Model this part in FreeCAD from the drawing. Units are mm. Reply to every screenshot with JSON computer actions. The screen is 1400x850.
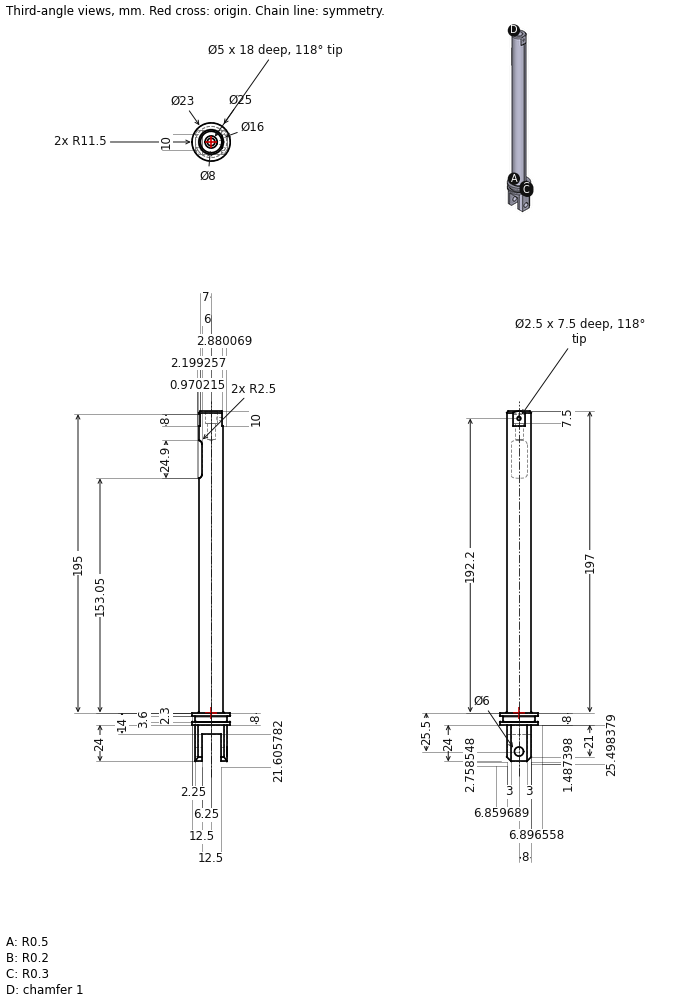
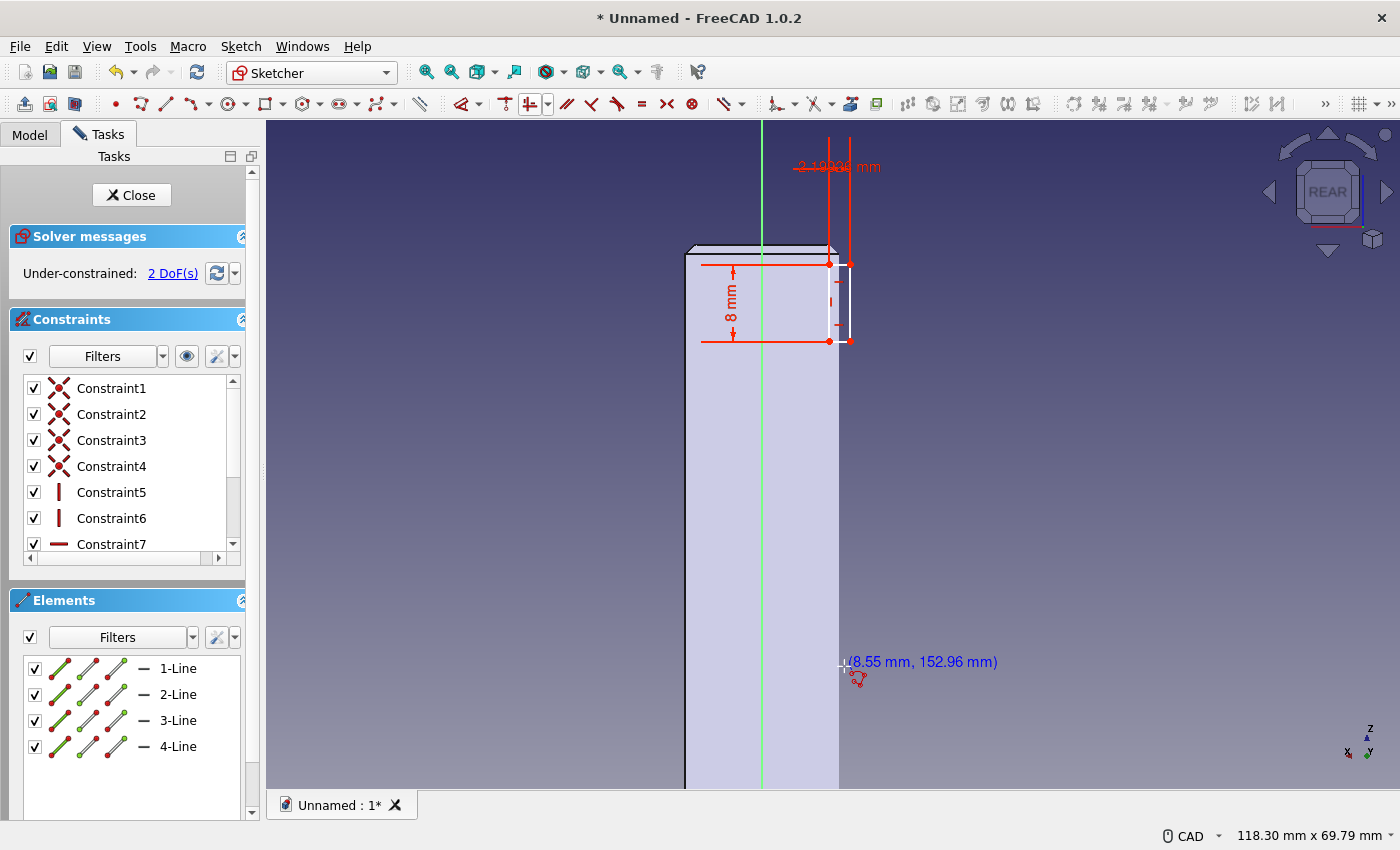
{"action": "scroll", "coordinate": [853, 666], "scroll_direction": "up", "scroll_amount": 3}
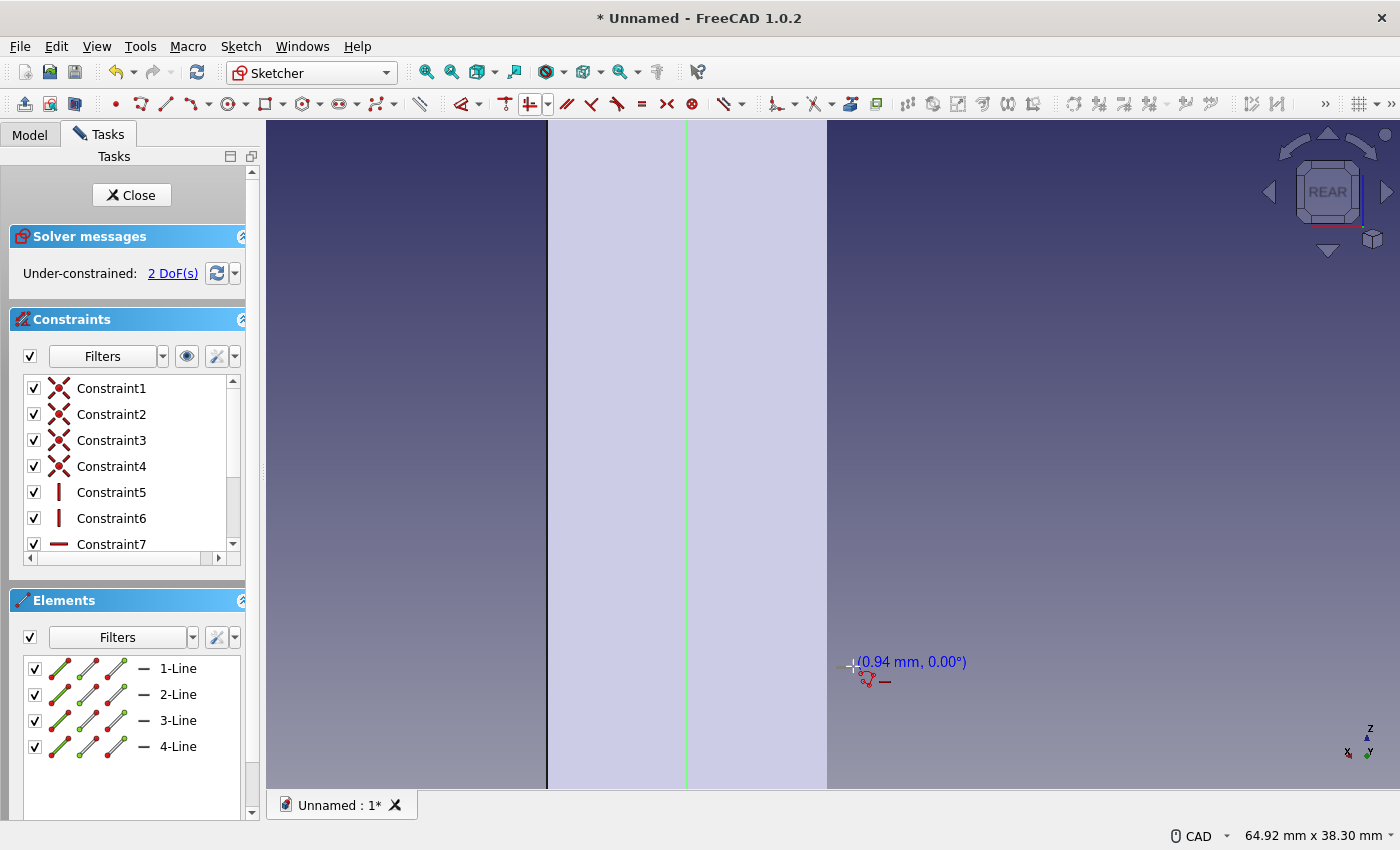
{"action": "left_click", "coordinate": [852, 665]}
{"action": "left_click", "coordinate": [852, 231]}
{"action": "left_click", "coordinate": [835, 231]}
{"action": "right_click", "coordinate": [835, 231]}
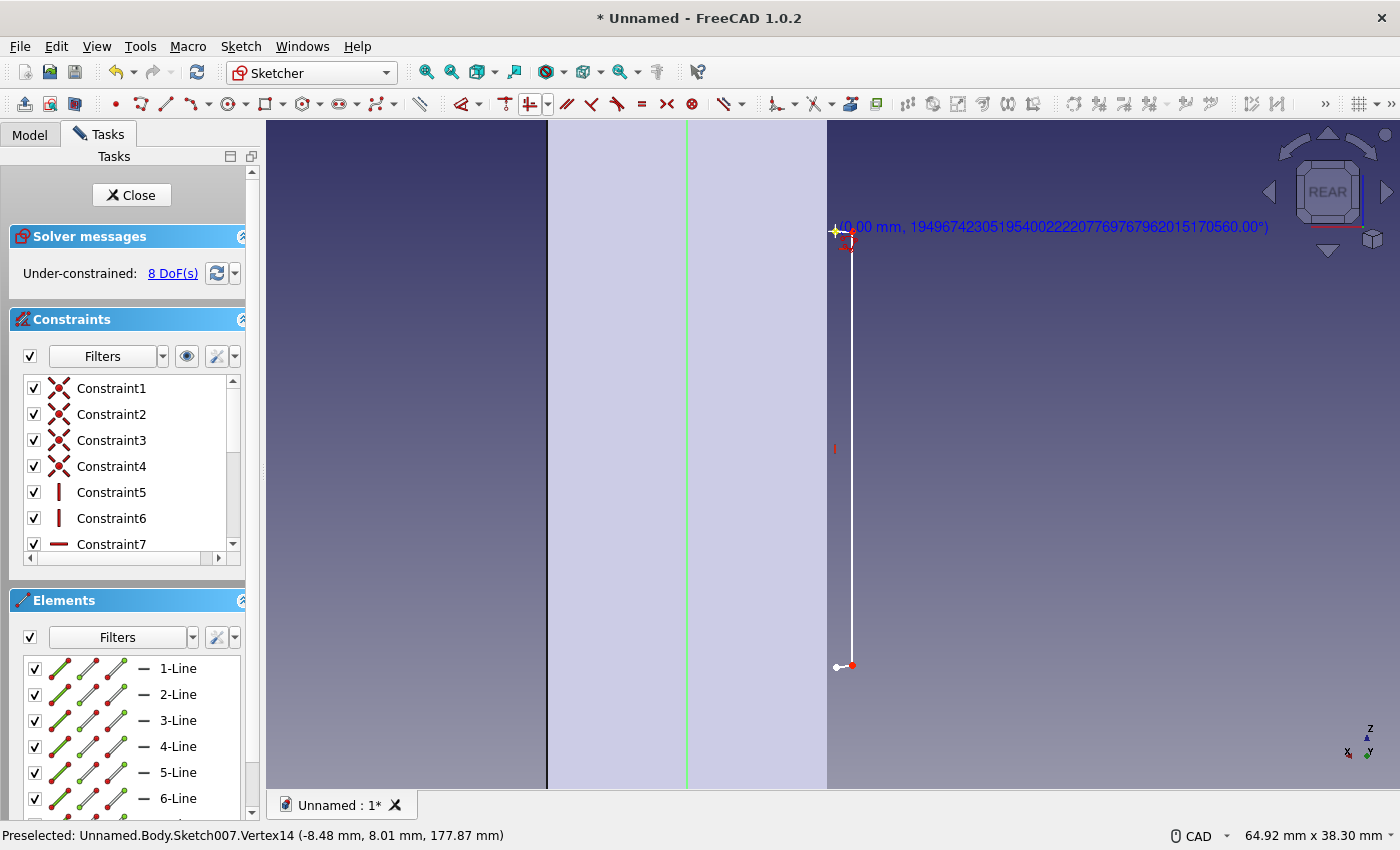
{"action": "left_click", "coordinate": [166, 104]}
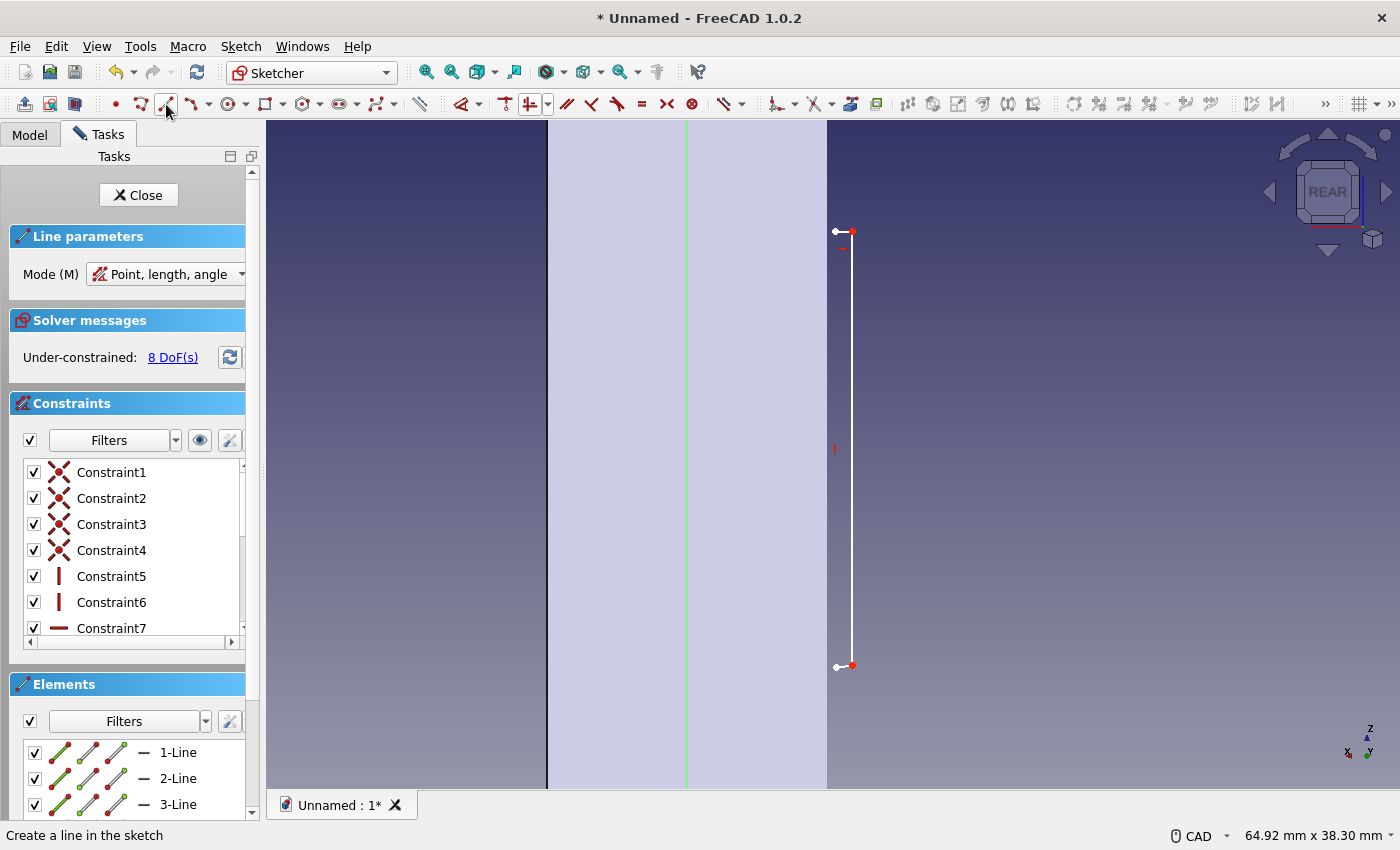
{"action": "left_click", "coordinate": [792, 274]}
{"action": "left_click", "coordinate": [792, 622]}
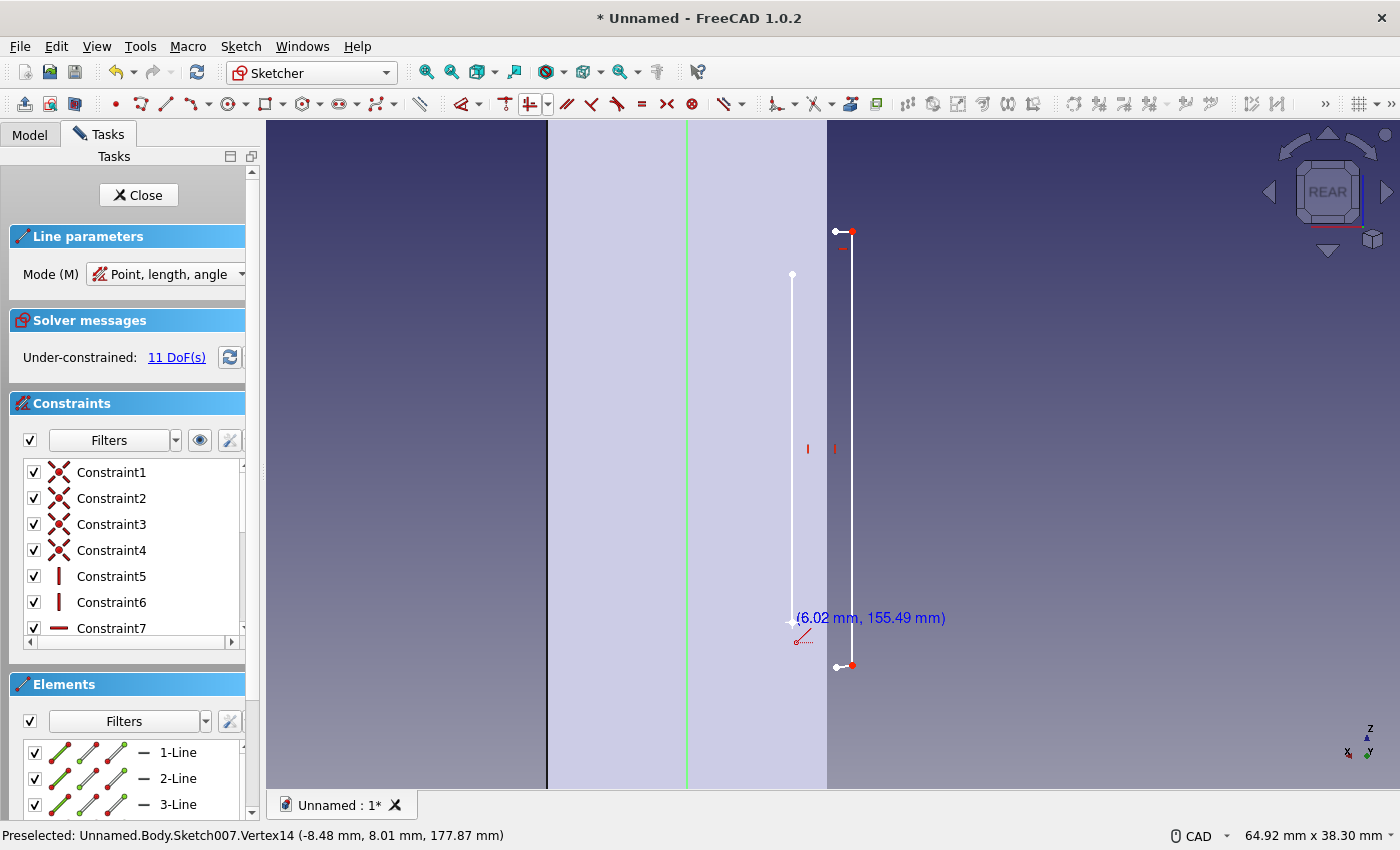
{"action": "left_click", "coordinate": [190, 104]}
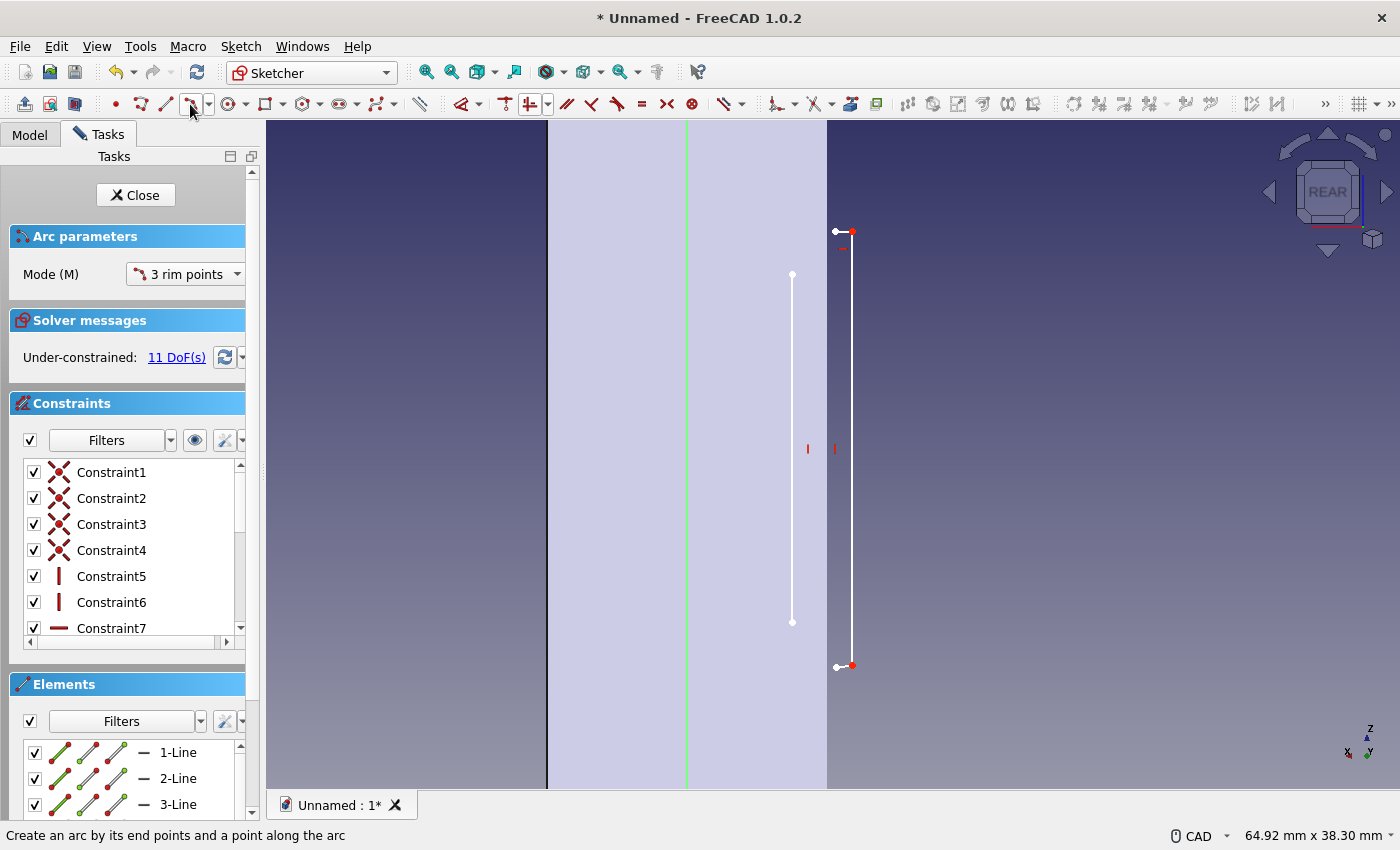
{"action": "scroll", "coordinate": [835, 231], "scroll_direction": "up", "scroll_amount": 4}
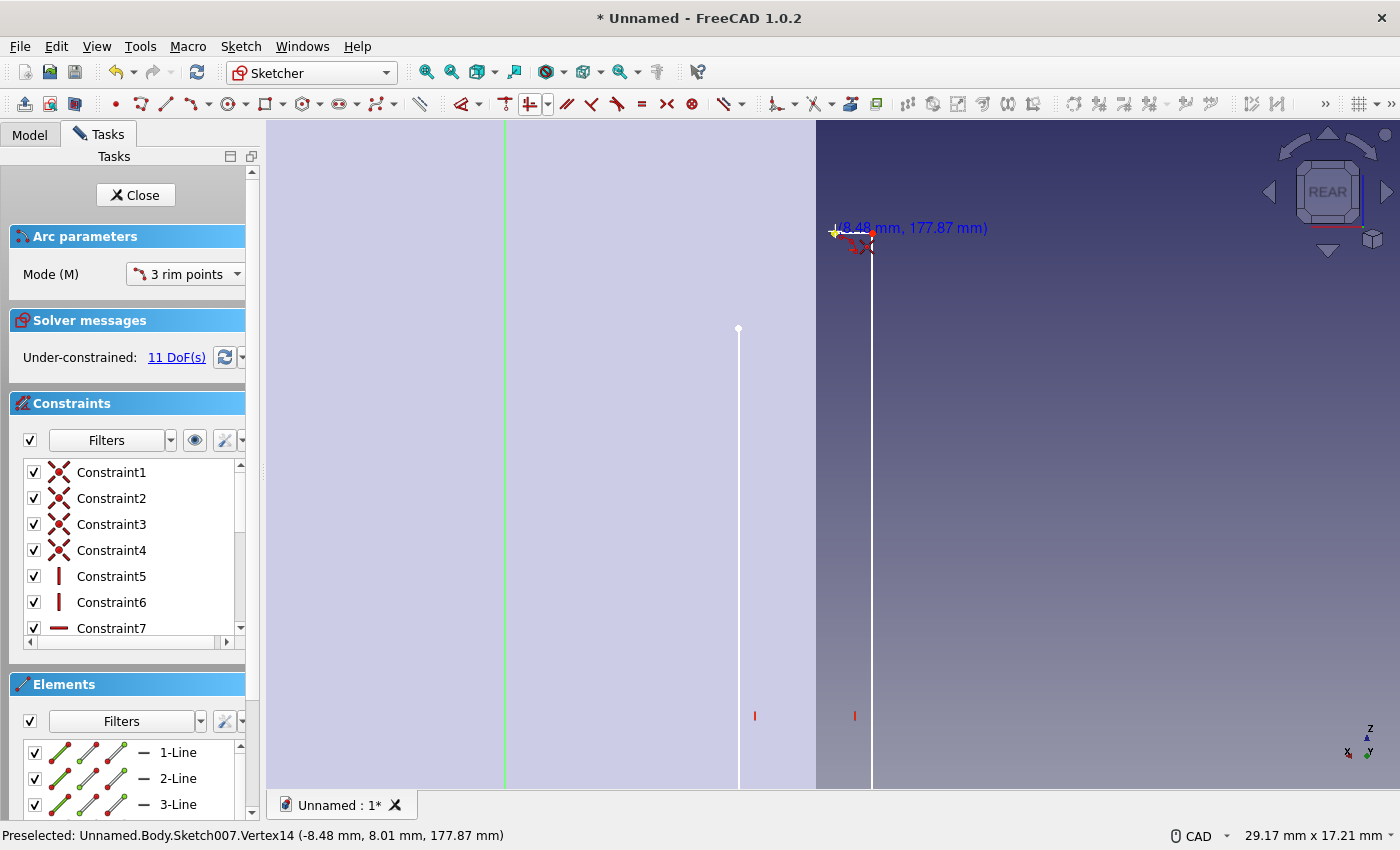
{"action": "left_click", "coordinate": [834, 233]}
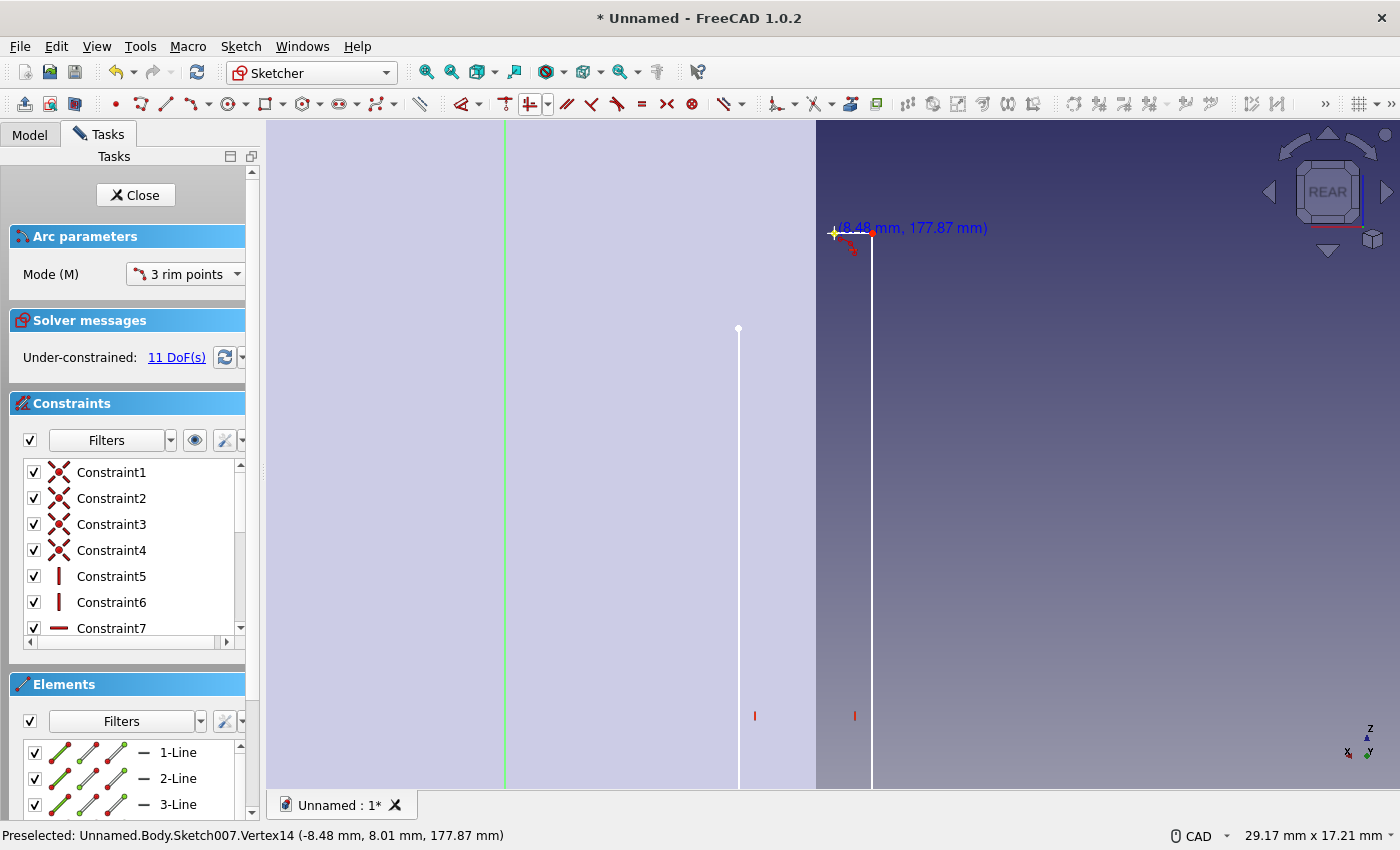
{"action": "scroll", "coordinate": [852, 491], "scroll_direction": "down", "scroll_amount": 7}